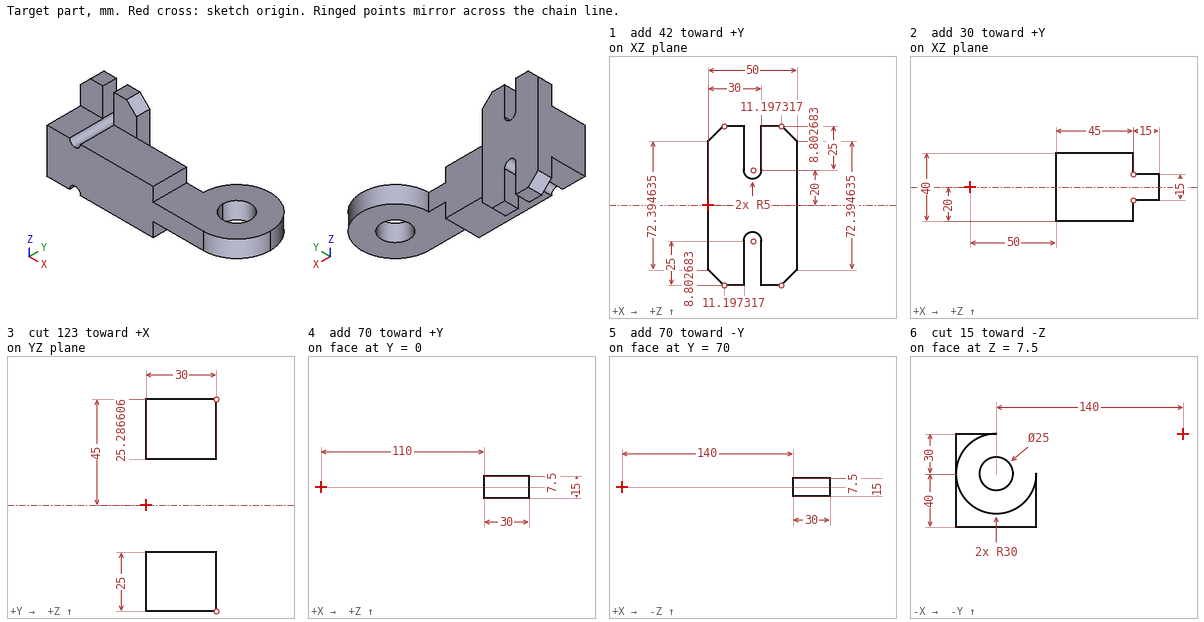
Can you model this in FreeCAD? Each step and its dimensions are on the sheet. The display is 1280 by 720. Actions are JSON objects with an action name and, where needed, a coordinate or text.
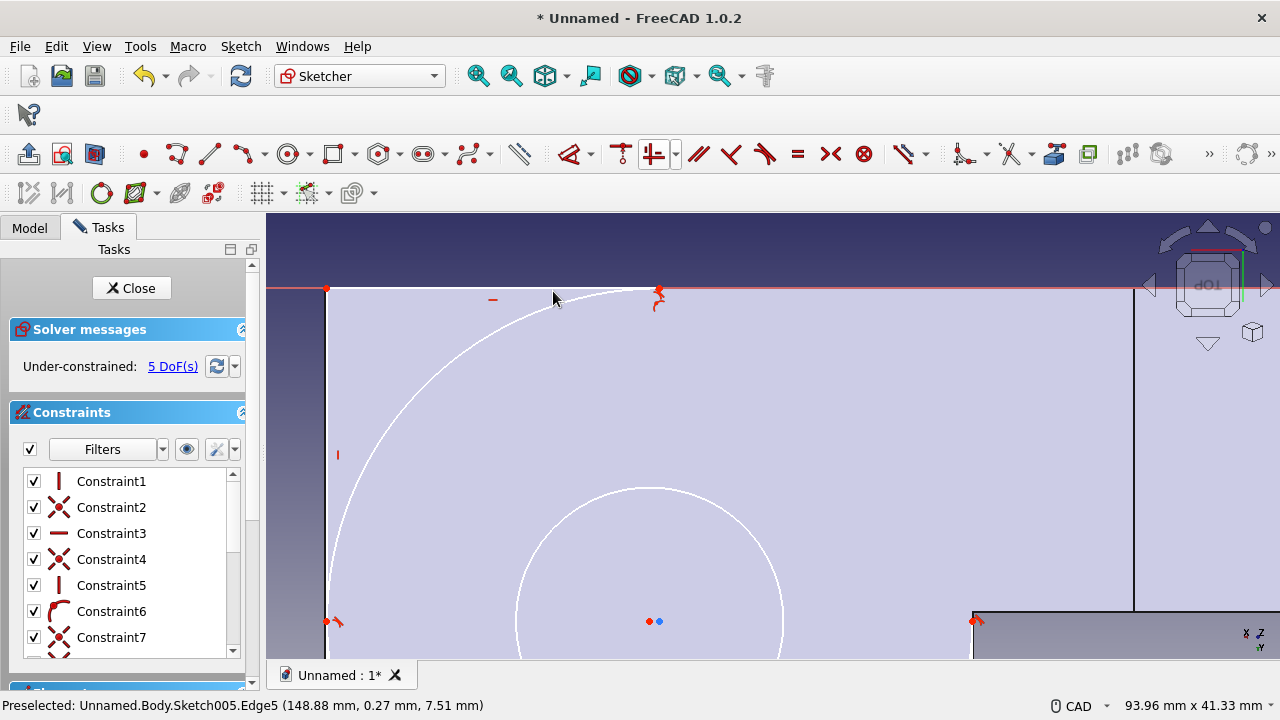
{"action": "left_click", "coordinate": [568, 154]}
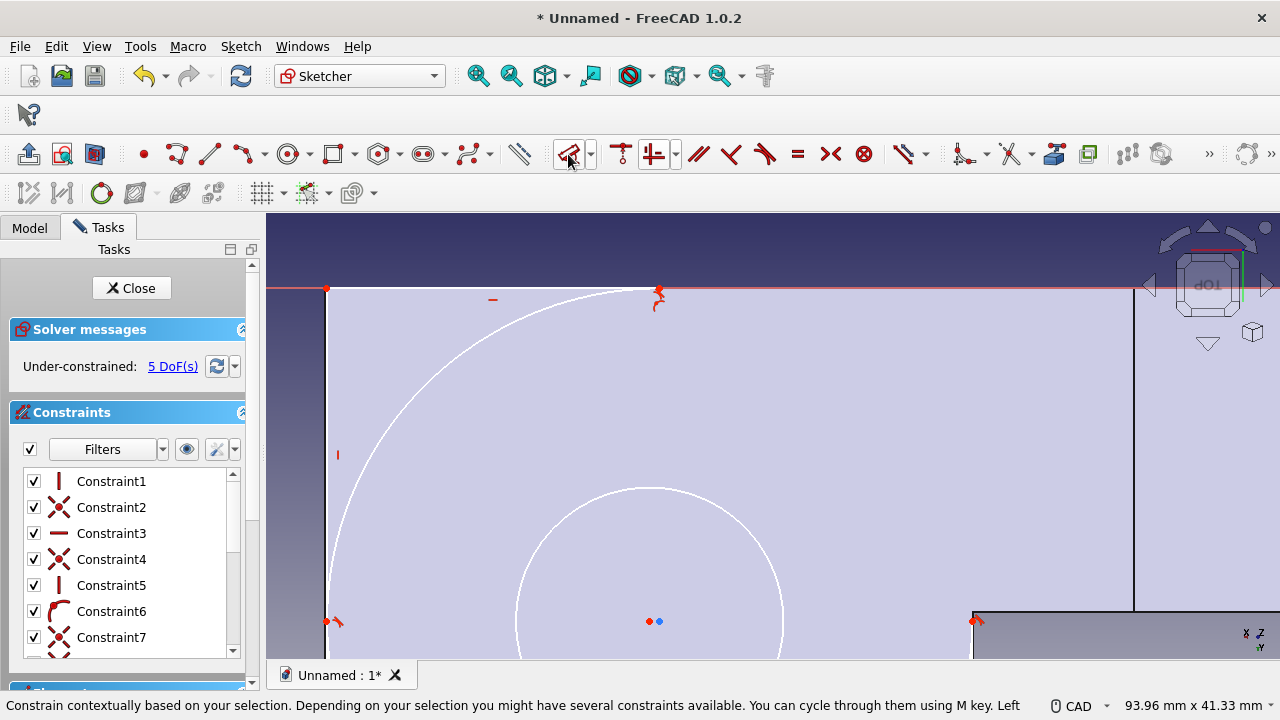
{"action": "scroll", "coordinate": [473, 337], "scroll_direction": "down", "scroll_amount": 6}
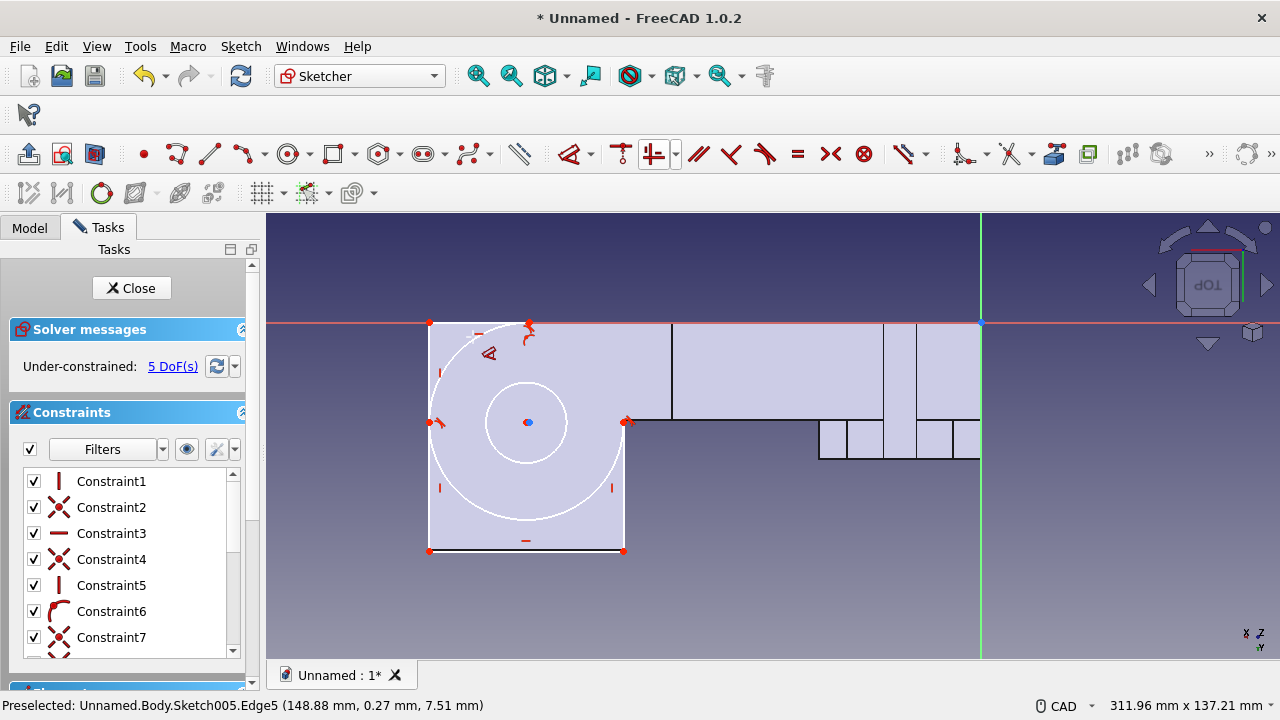
{"action": "left_click", "coordinate": [469, 501]}
{"action": "left_click", "coordinate": [450, 527]}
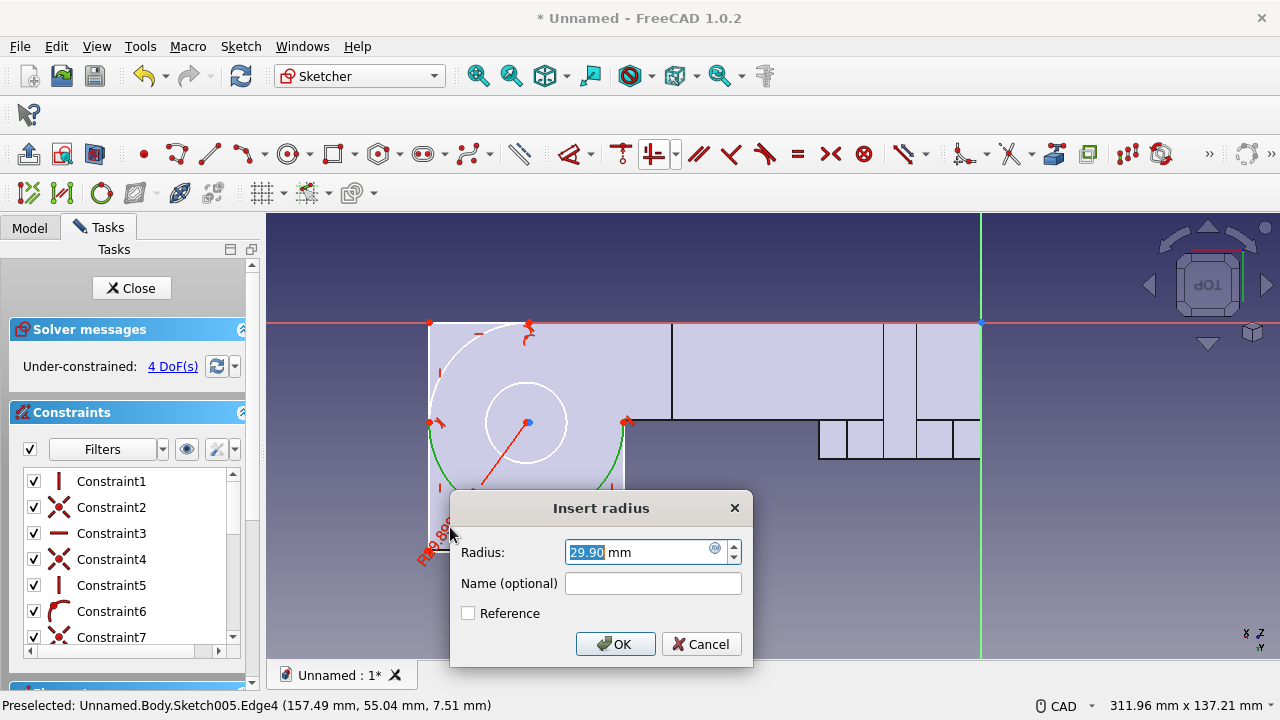
{"action": "type", "text": "30"}
{"action": "key", "text": "Return"}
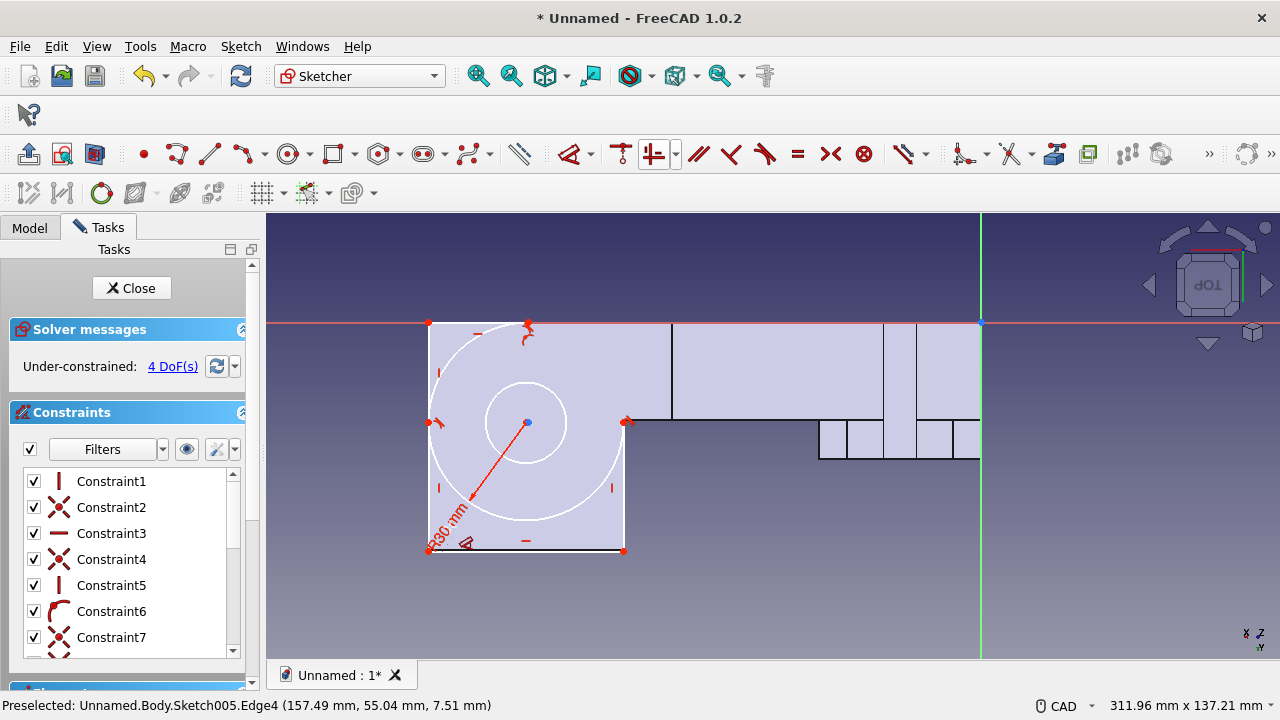
{"action": "left_click", "coordinate": [554, 394]}
{"action": "left_click", "coordinate": [576, 371]}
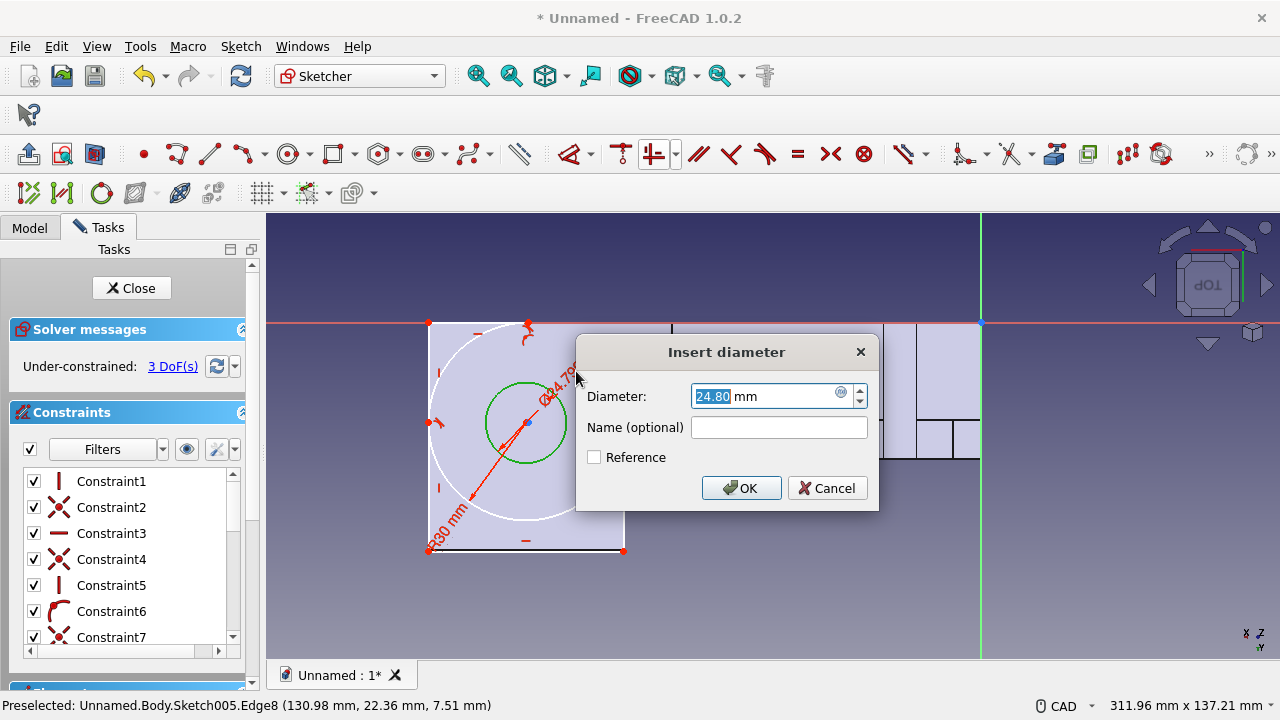
{"action": "type", "text": "25"}
{"action": "key", "text": "Return"}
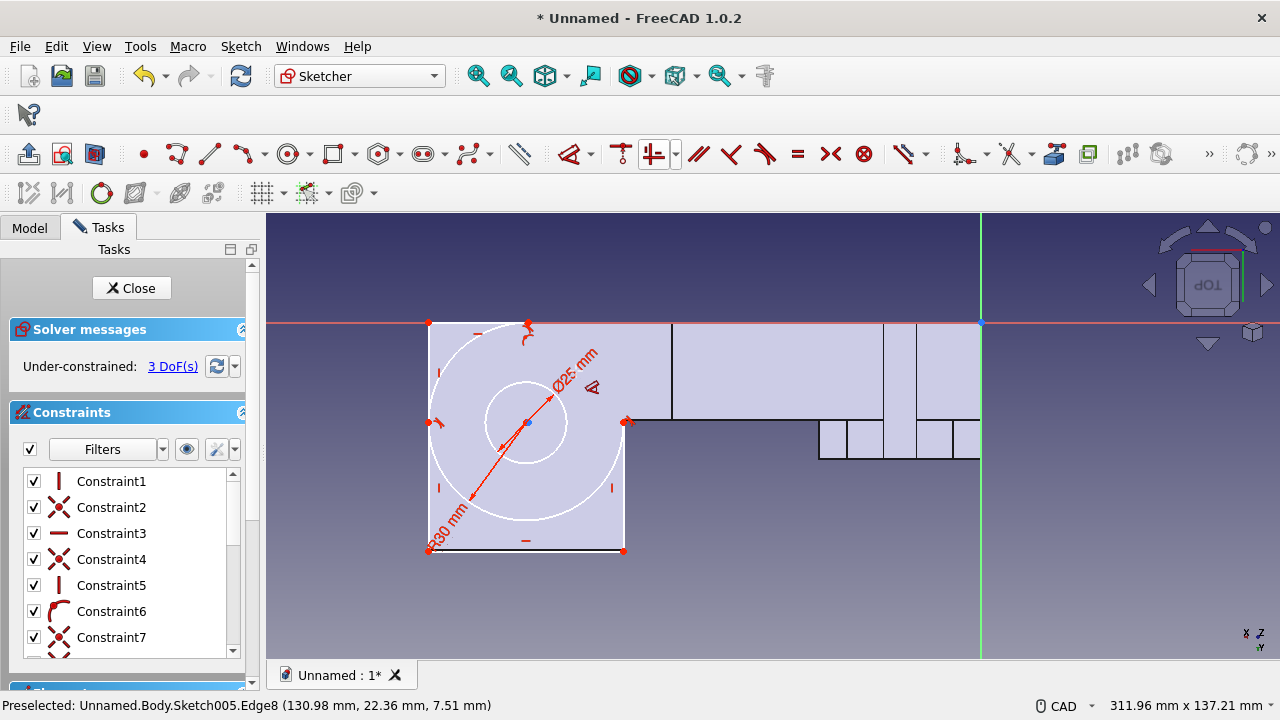
{"action": "left_click", "coordinate": [429, 513]}
{"action": "left_click", "coordinate": [395, 487]}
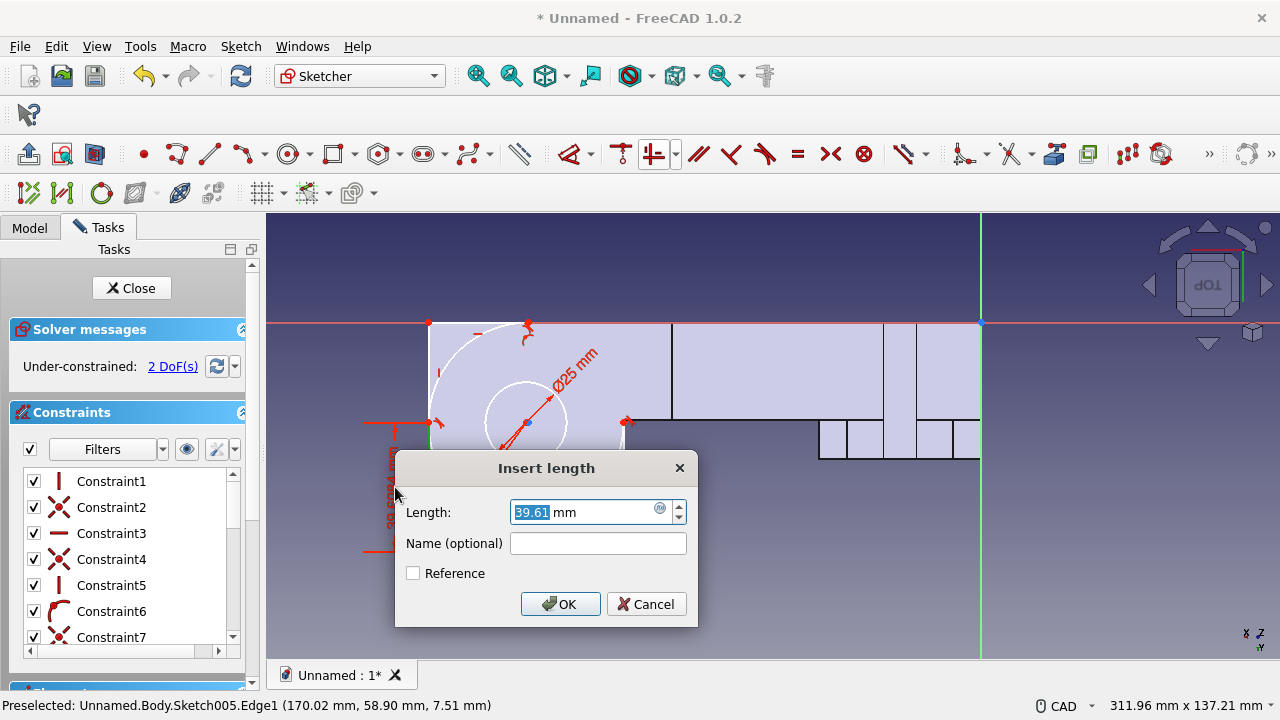
{"action": "type", "text": "40"}
{"action": "key", "text": "Return"}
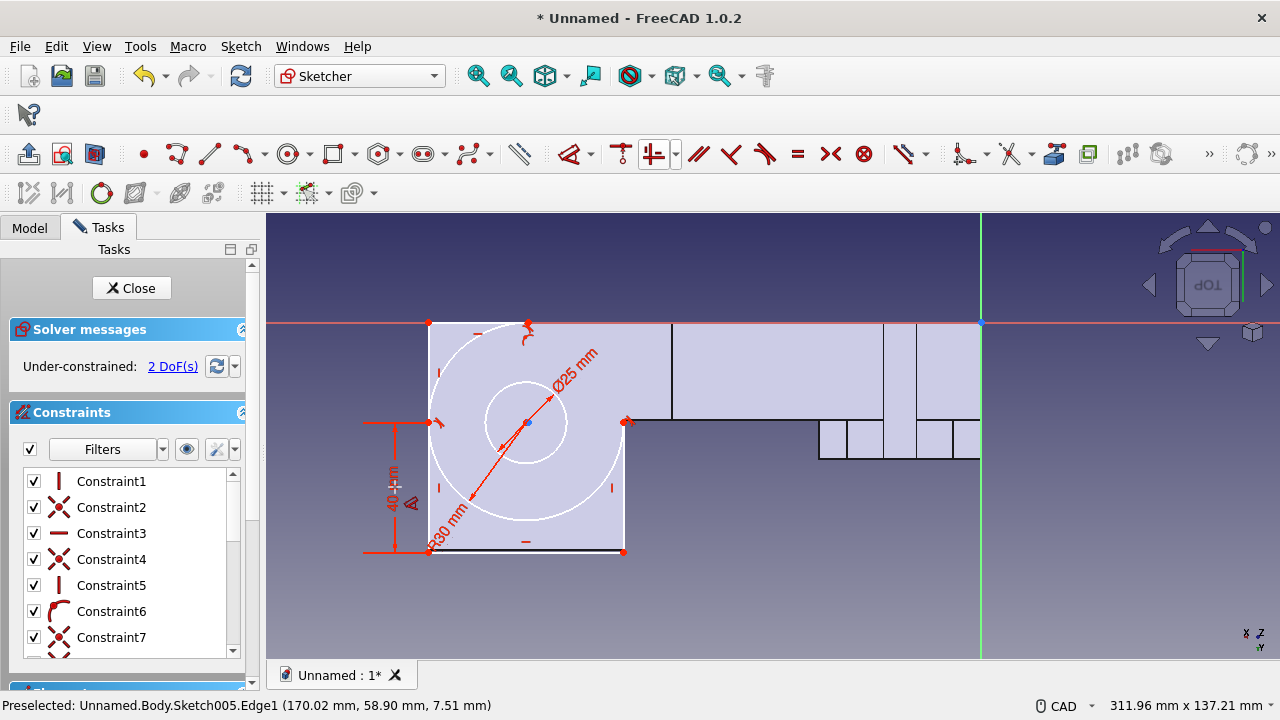
{"action": "left_click", "coordinate": [429, 353]}
{"action": "left_click", "coordinate": [395, 373]}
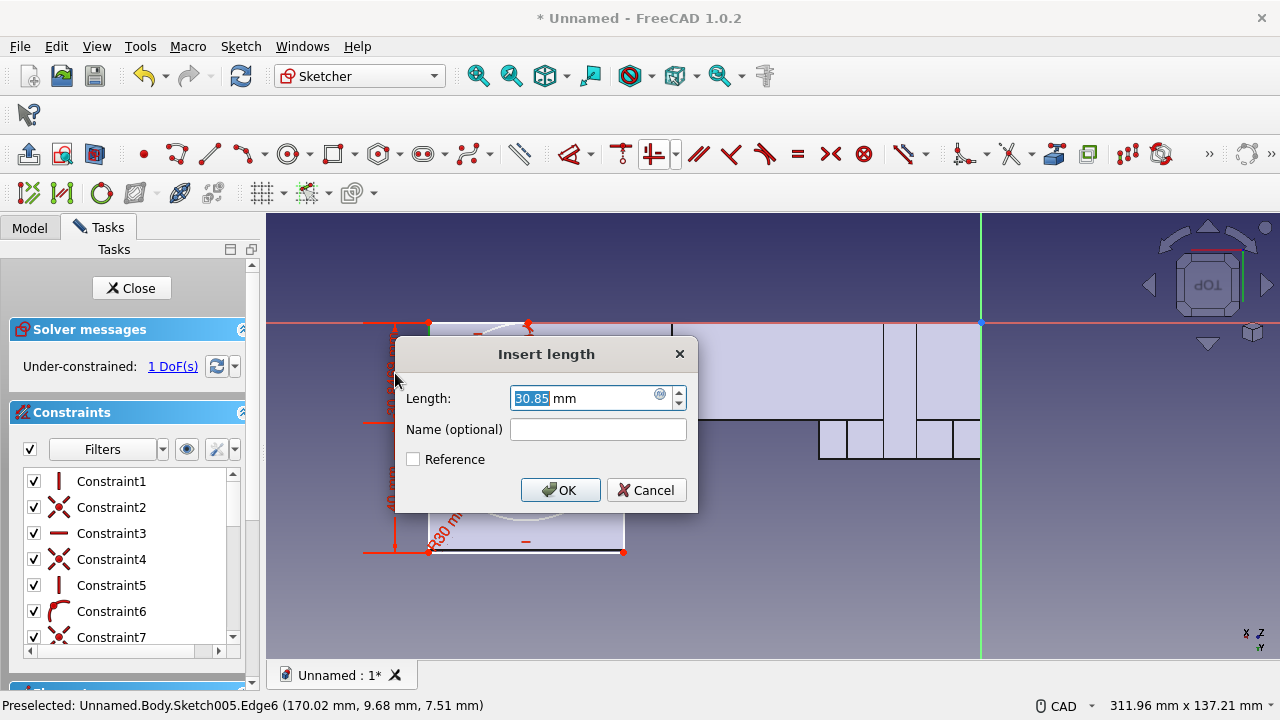
{"action": "type", "text": "30"}
{"action": "key", "text": "Return"}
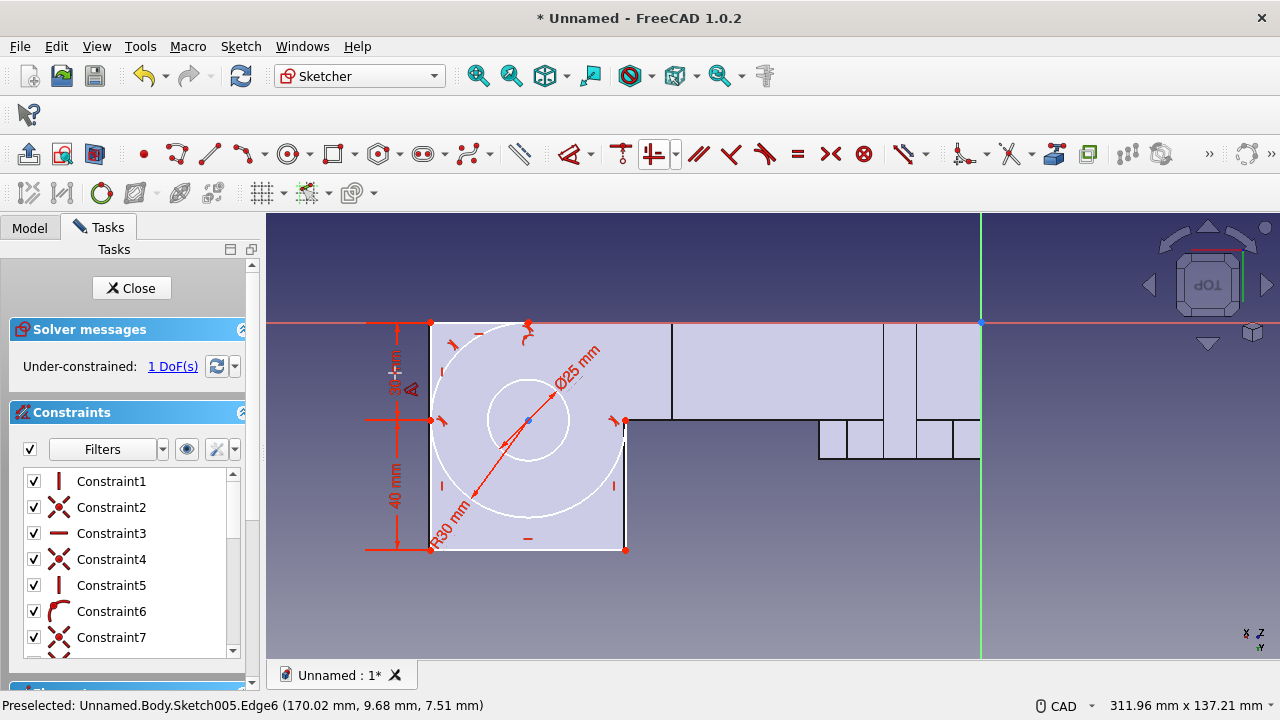
{"action": "left_click", "coordinate": [528, 420]}
{"action": "left_click", "coordinate": [755, 289]}